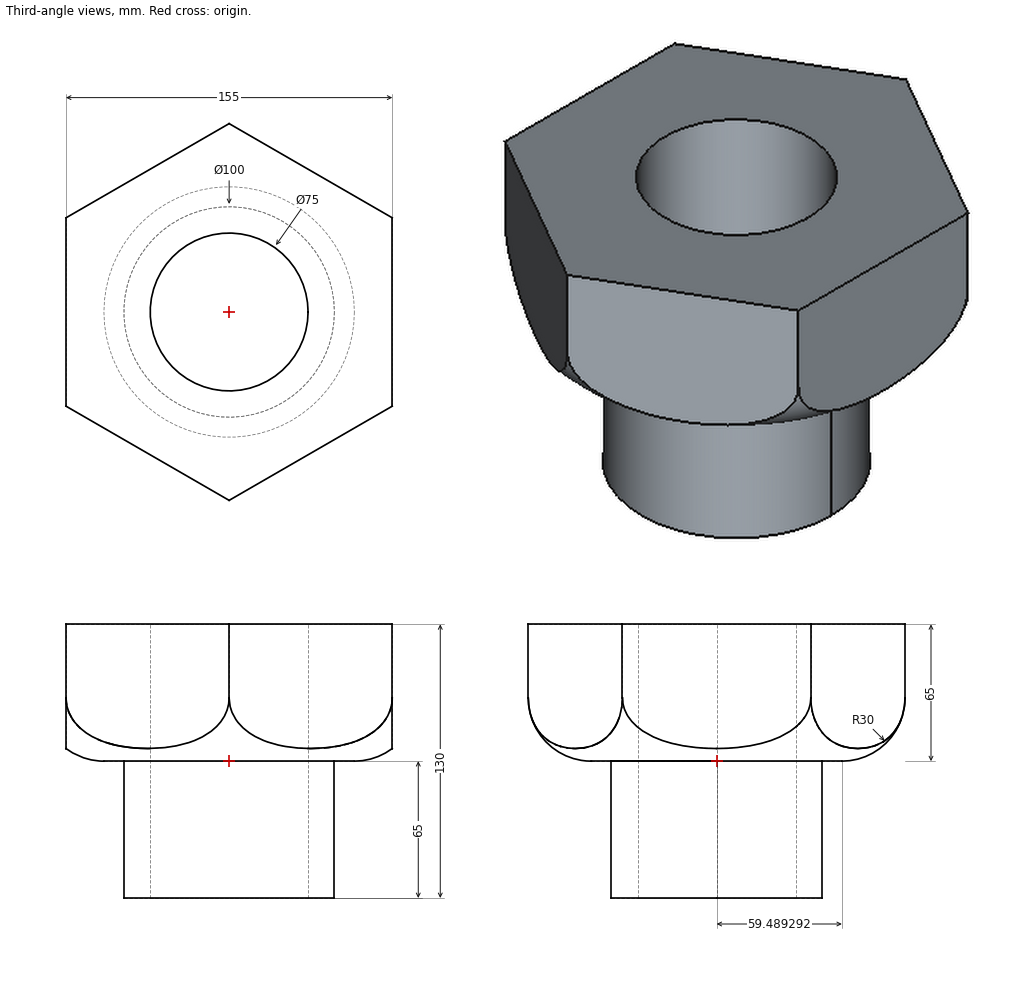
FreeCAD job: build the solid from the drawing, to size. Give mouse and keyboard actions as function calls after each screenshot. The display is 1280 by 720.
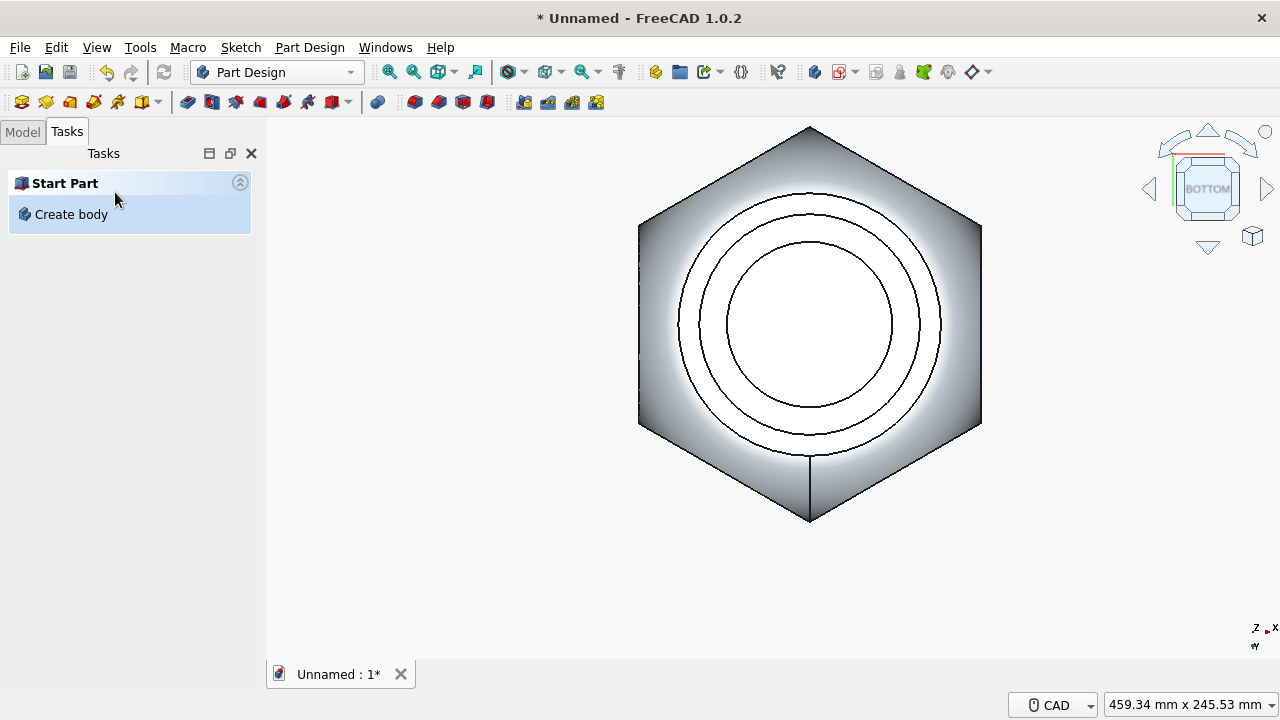
key(0)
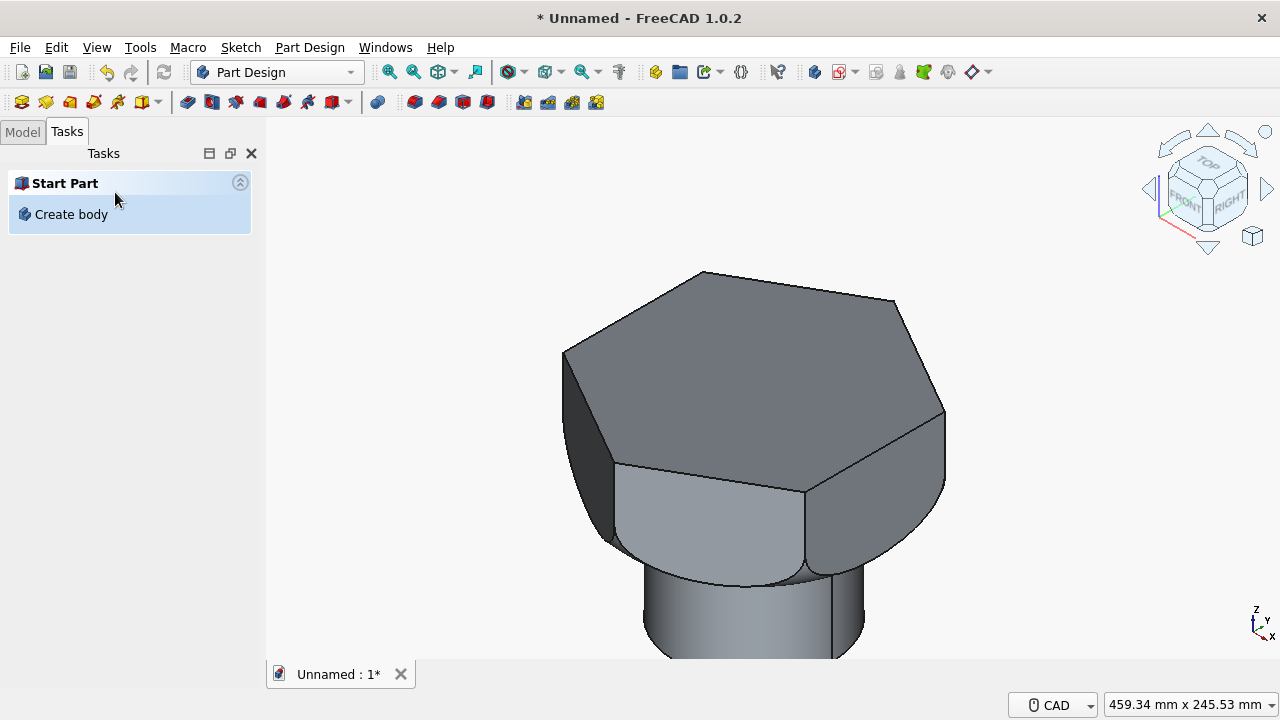
key(v)
key(f)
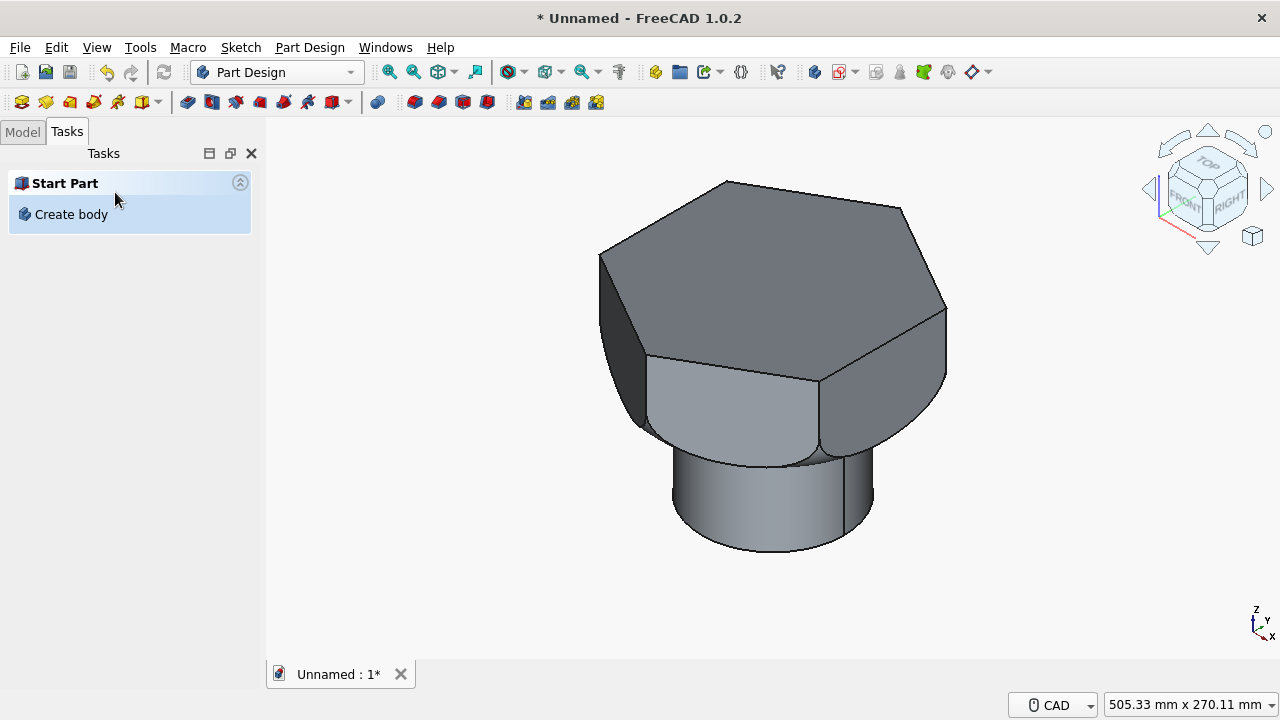
click(773, 281)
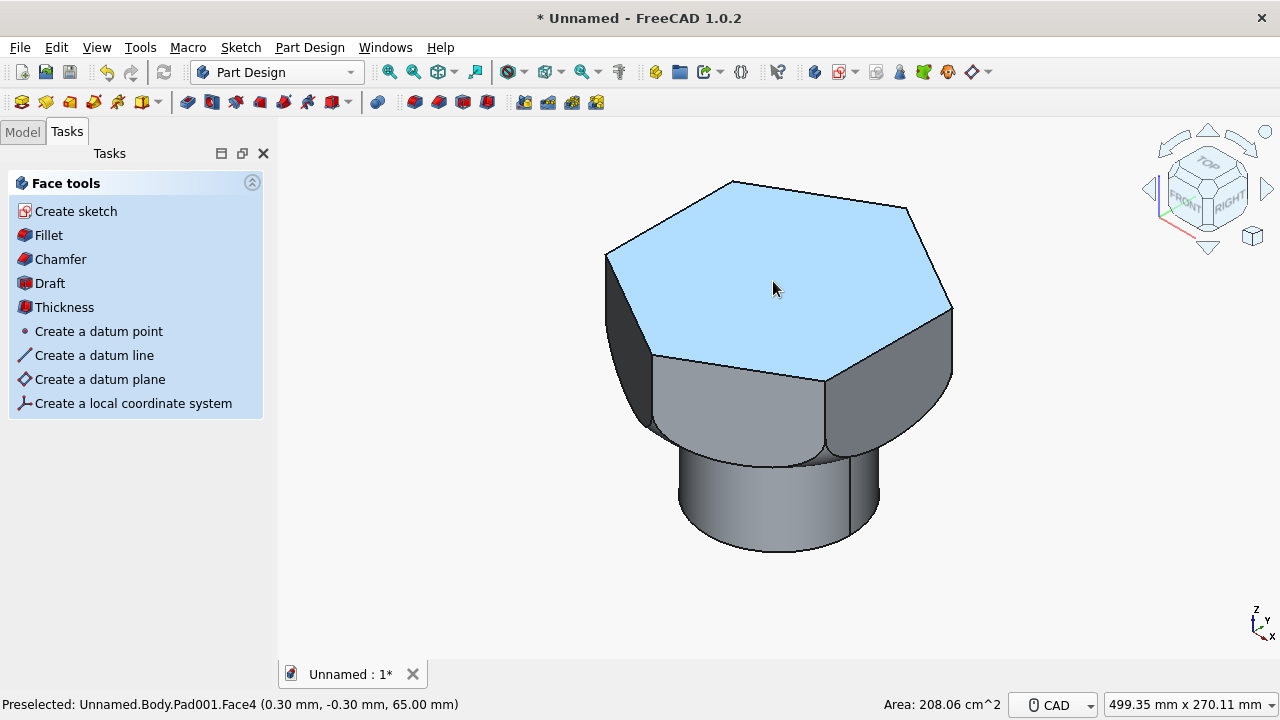
click(840, 72)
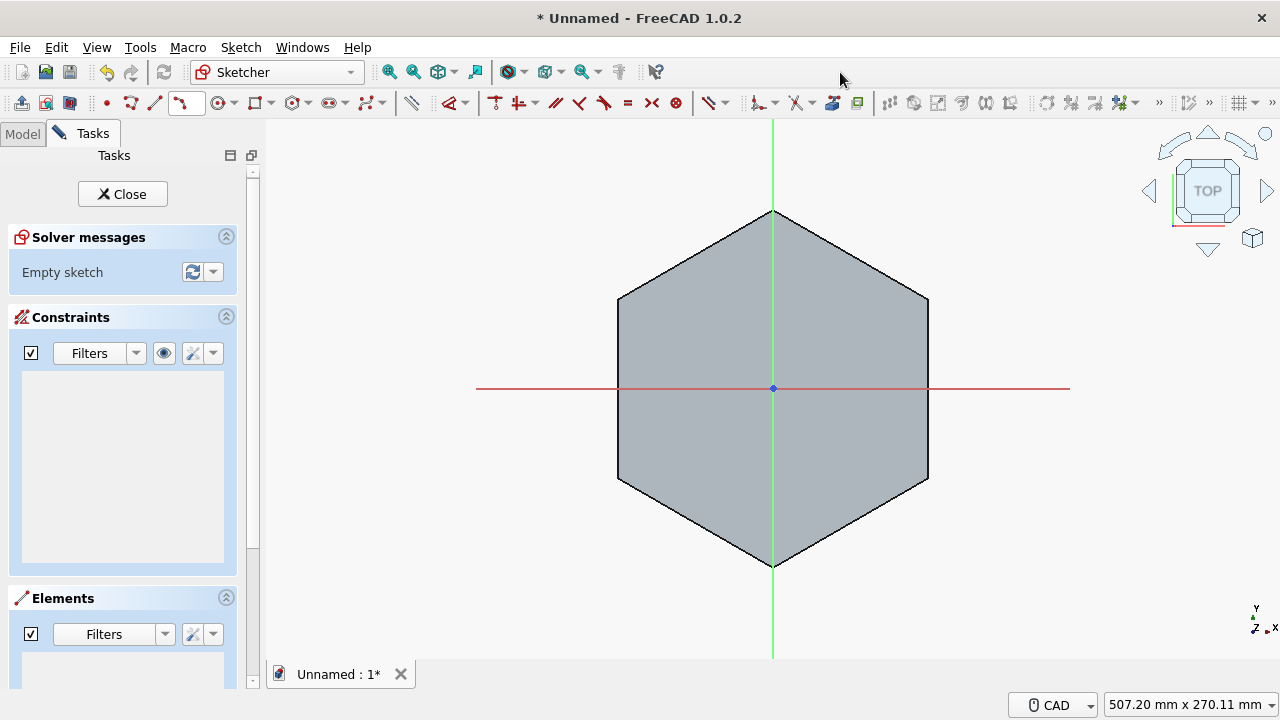
scroll(829, 389, up, 4)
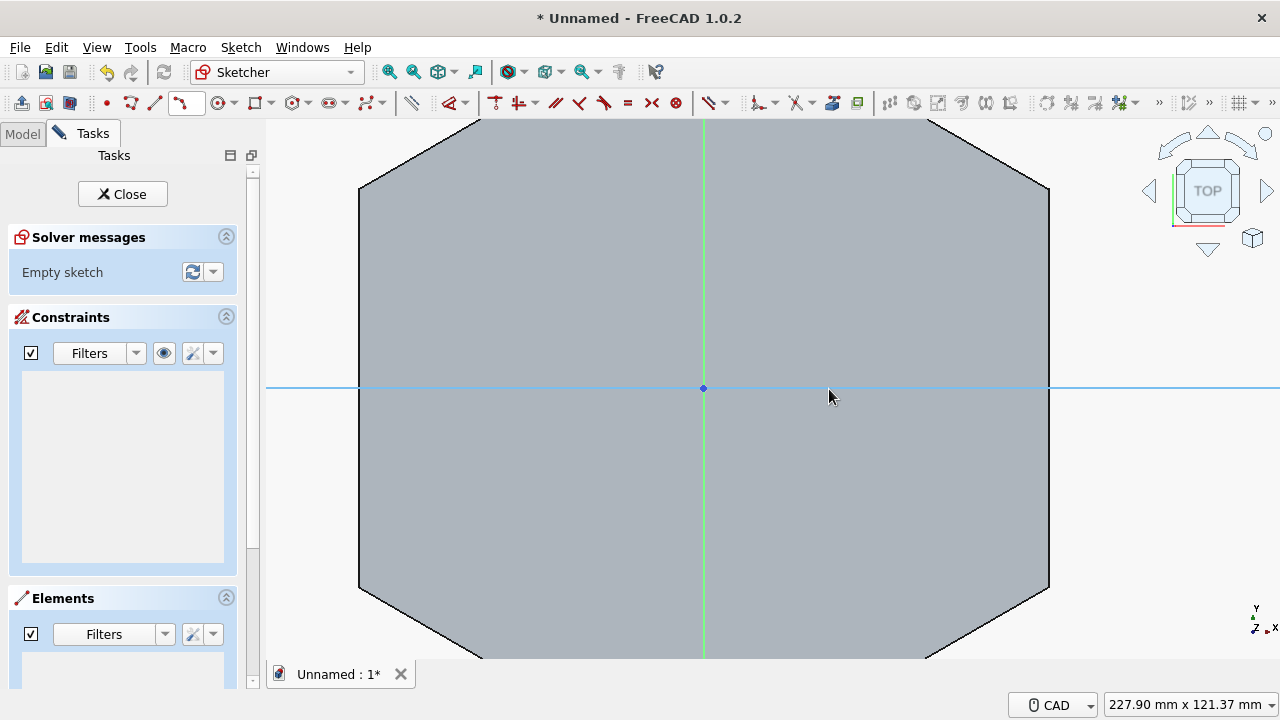
click(218, 104)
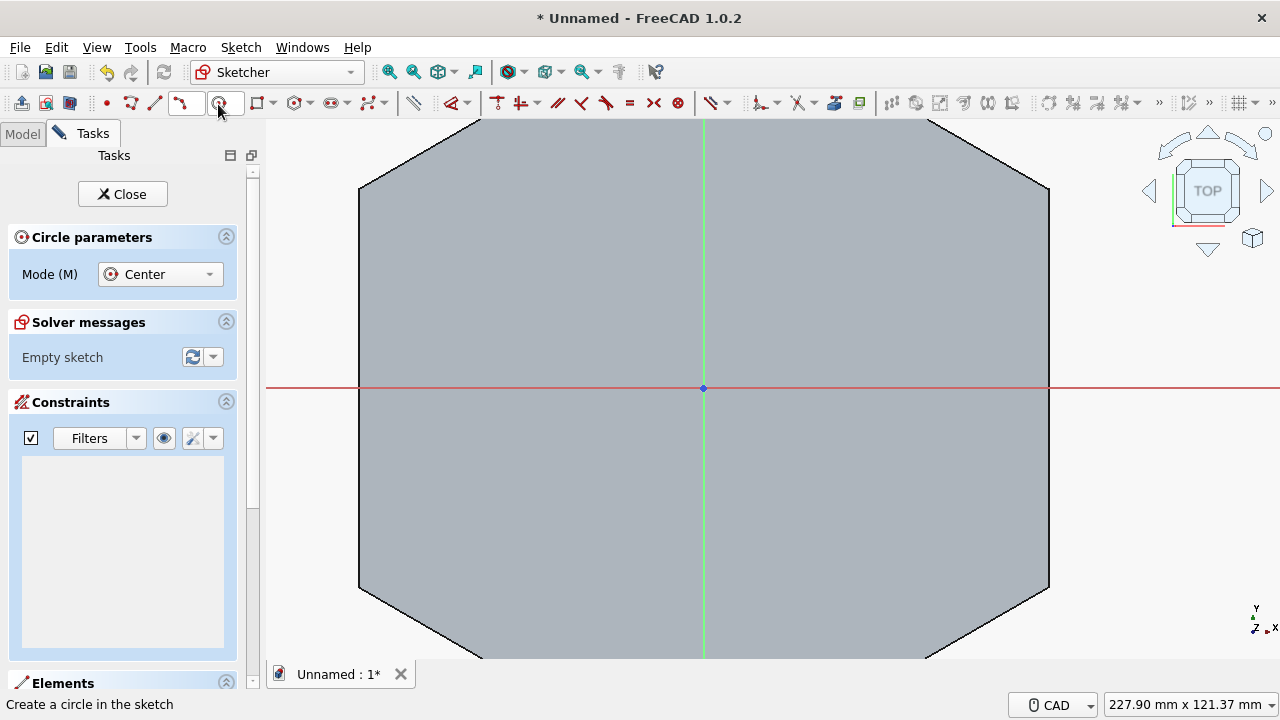
click(704, 388)
move(822, 270)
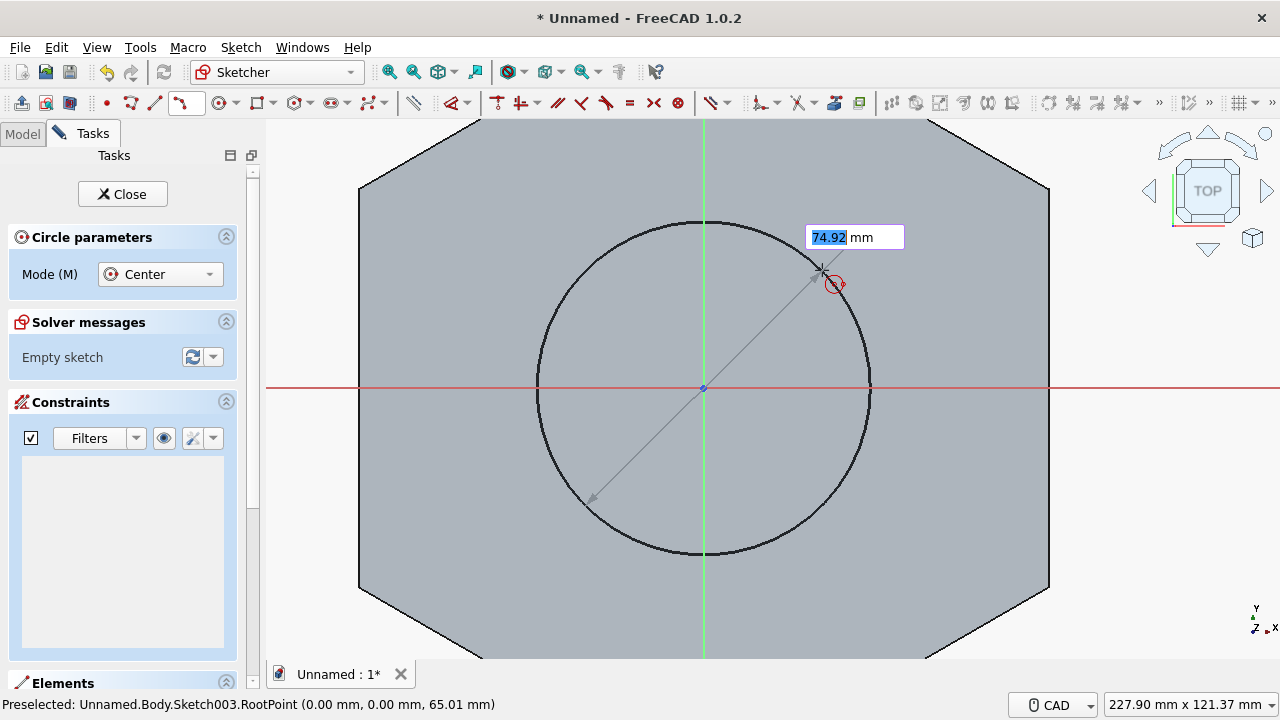
text(75)
key(Return)
key(Escape)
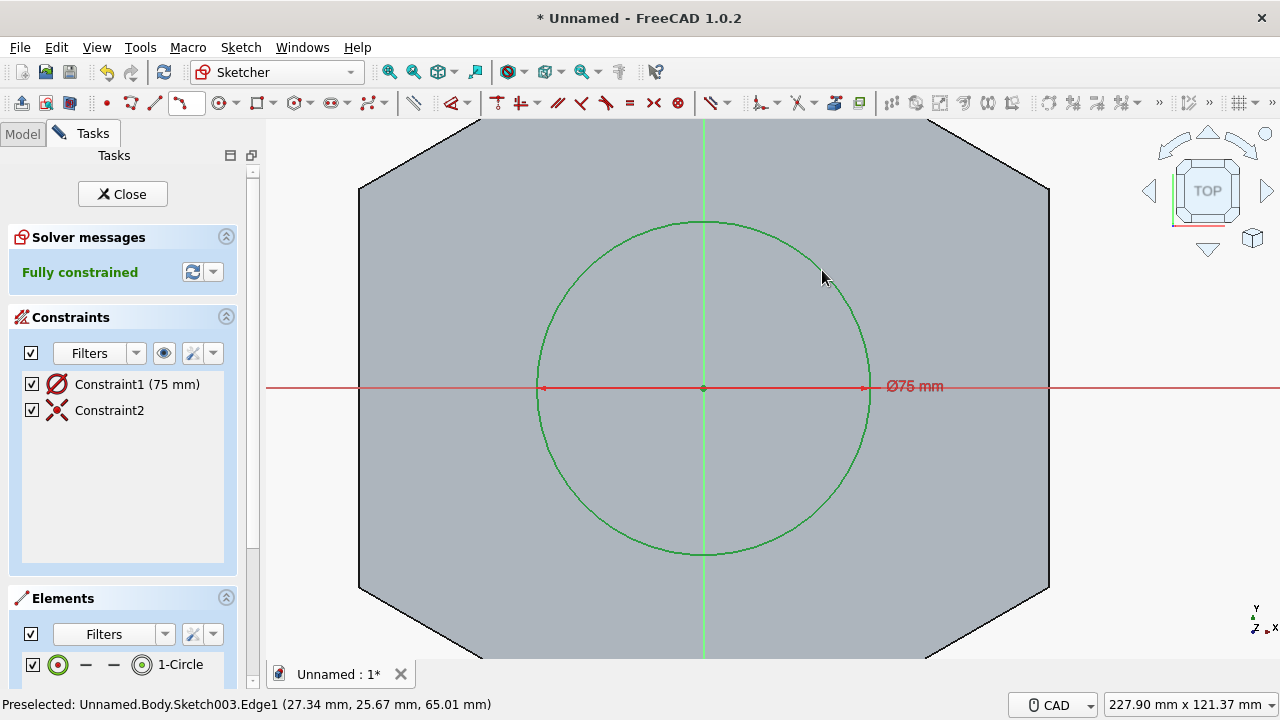
click(123, 194)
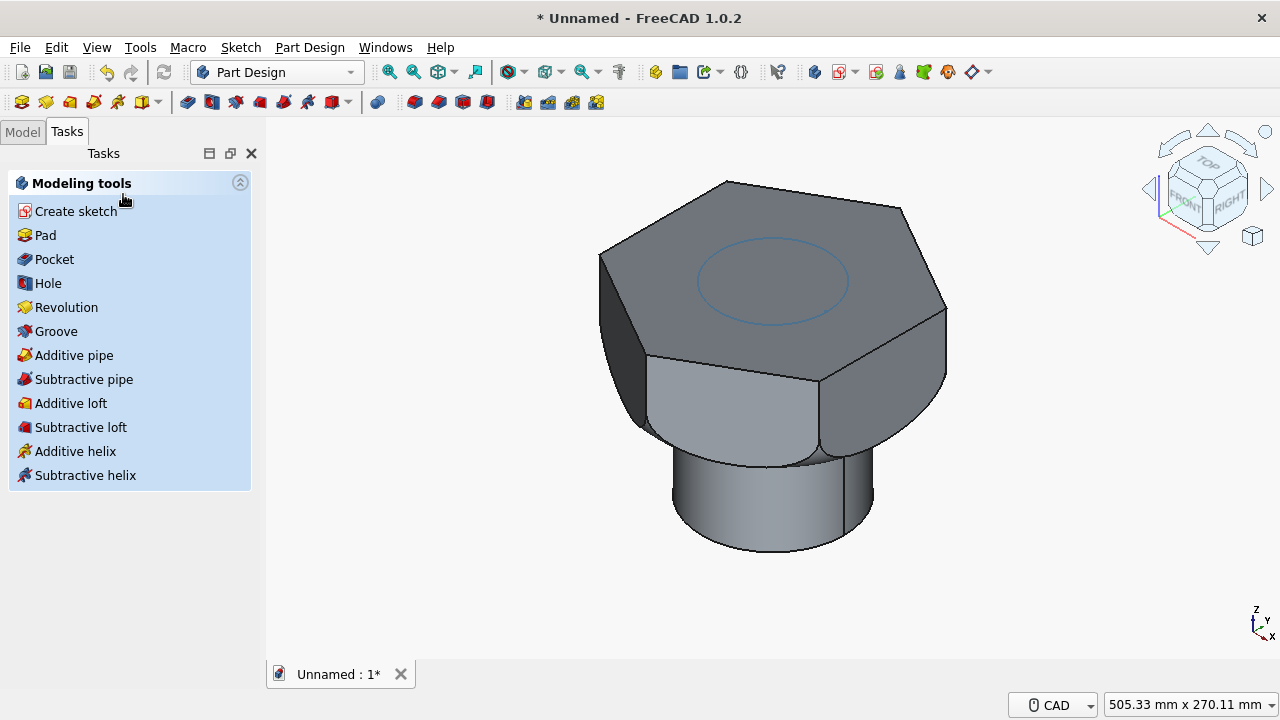
click(188, 102)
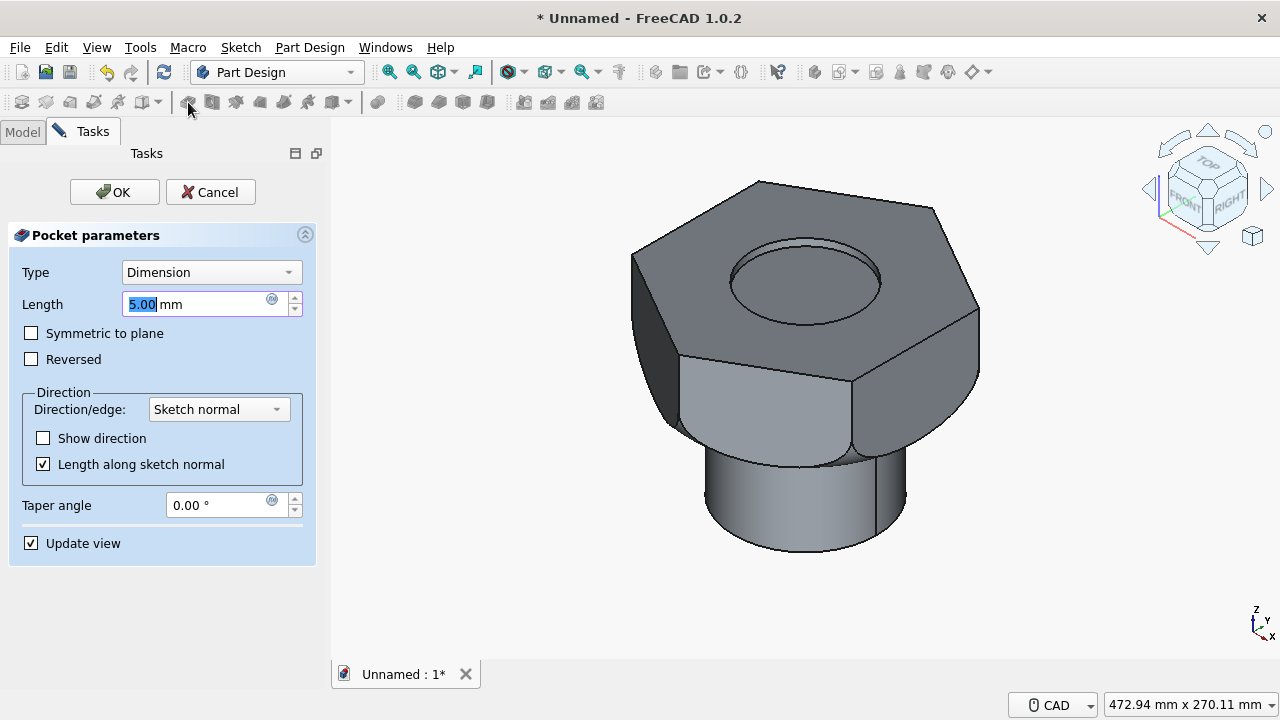
text(130)
key(Tab)